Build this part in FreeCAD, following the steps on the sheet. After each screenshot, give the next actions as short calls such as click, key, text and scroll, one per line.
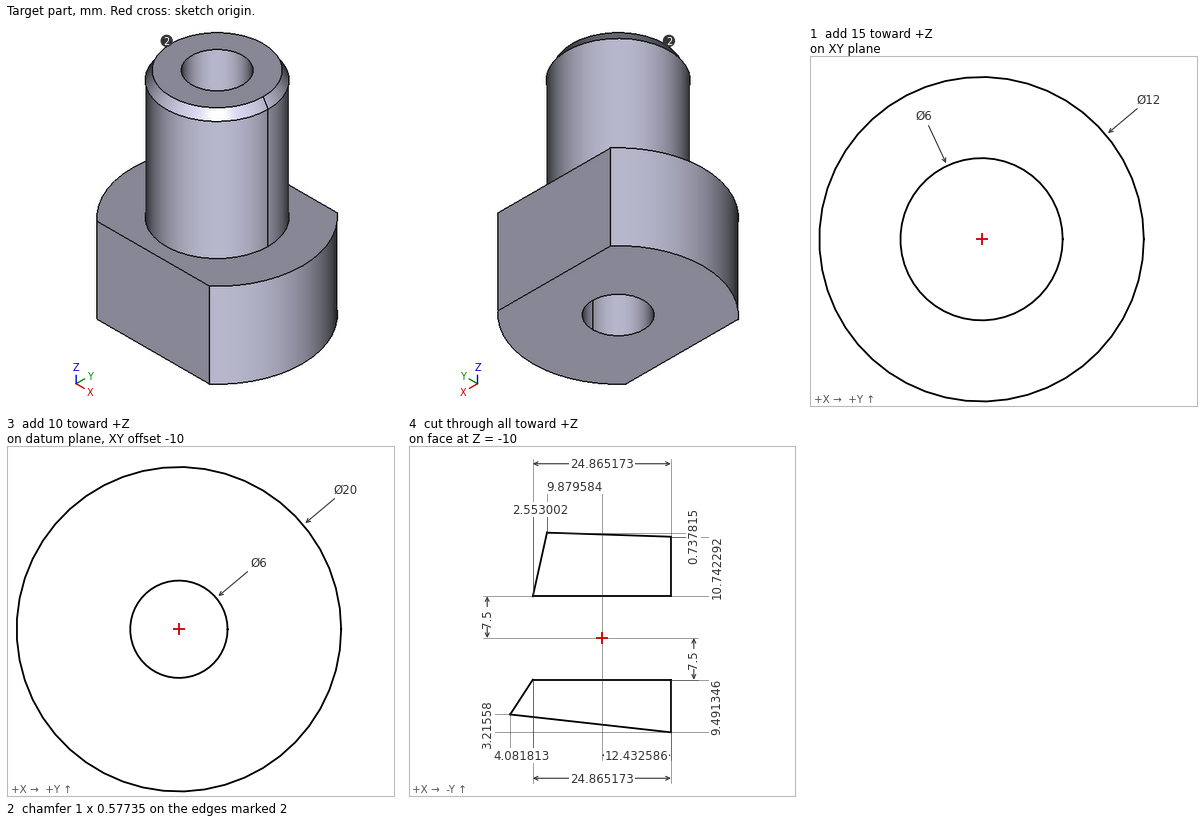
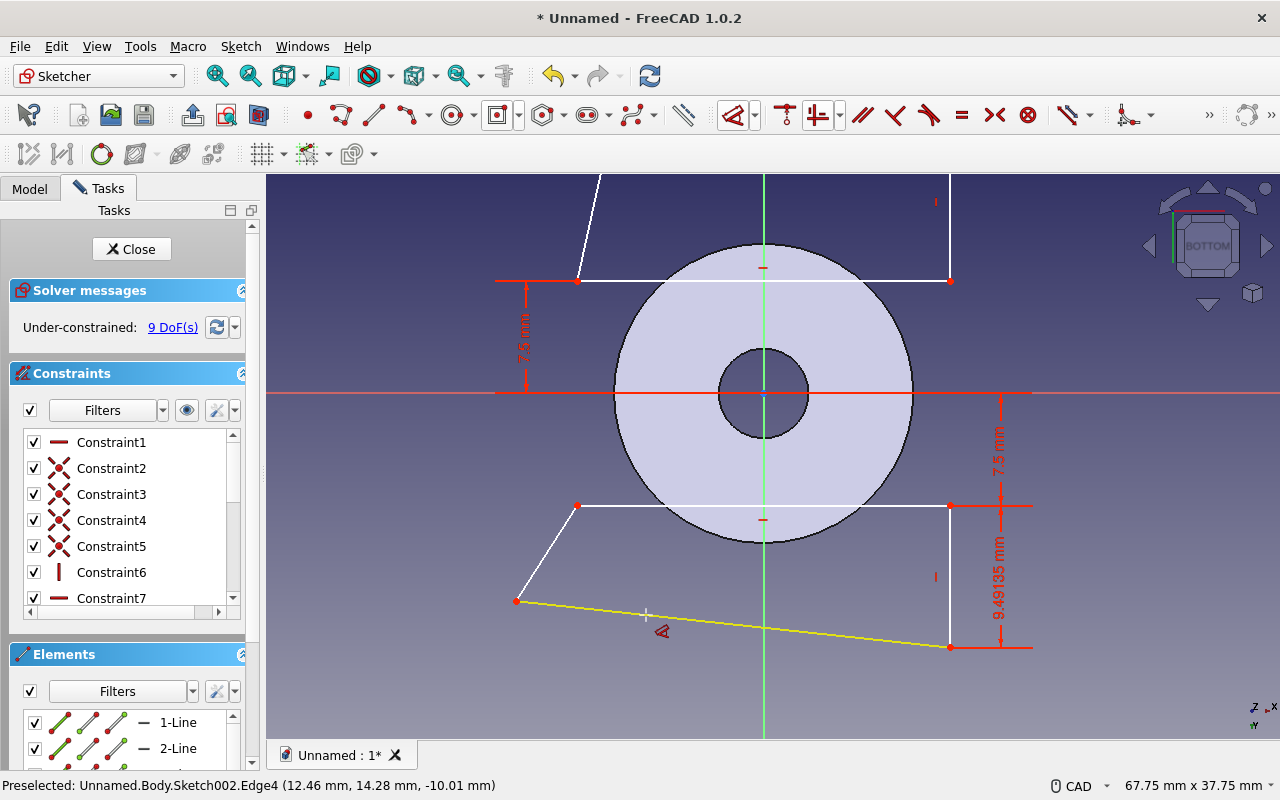
click(646, 615)
click(482, 624)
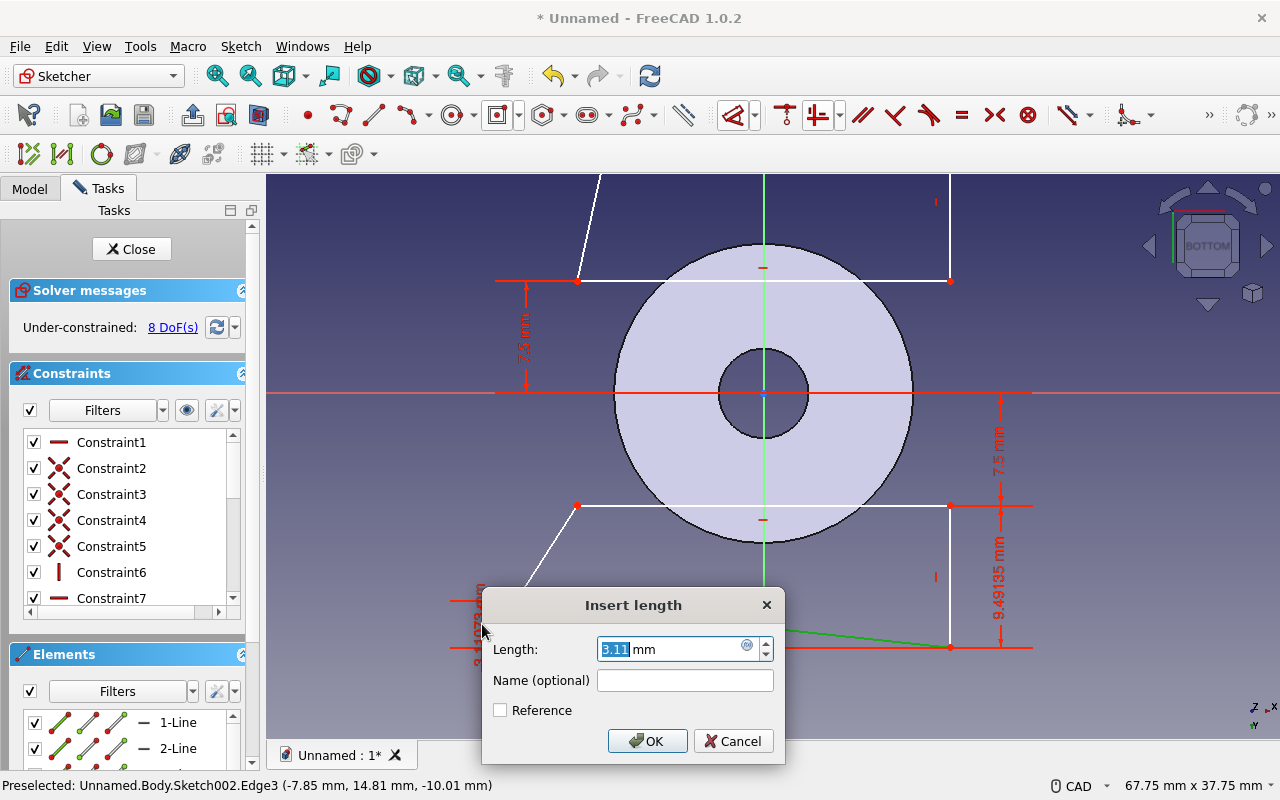
text(3.21558)
key(Return)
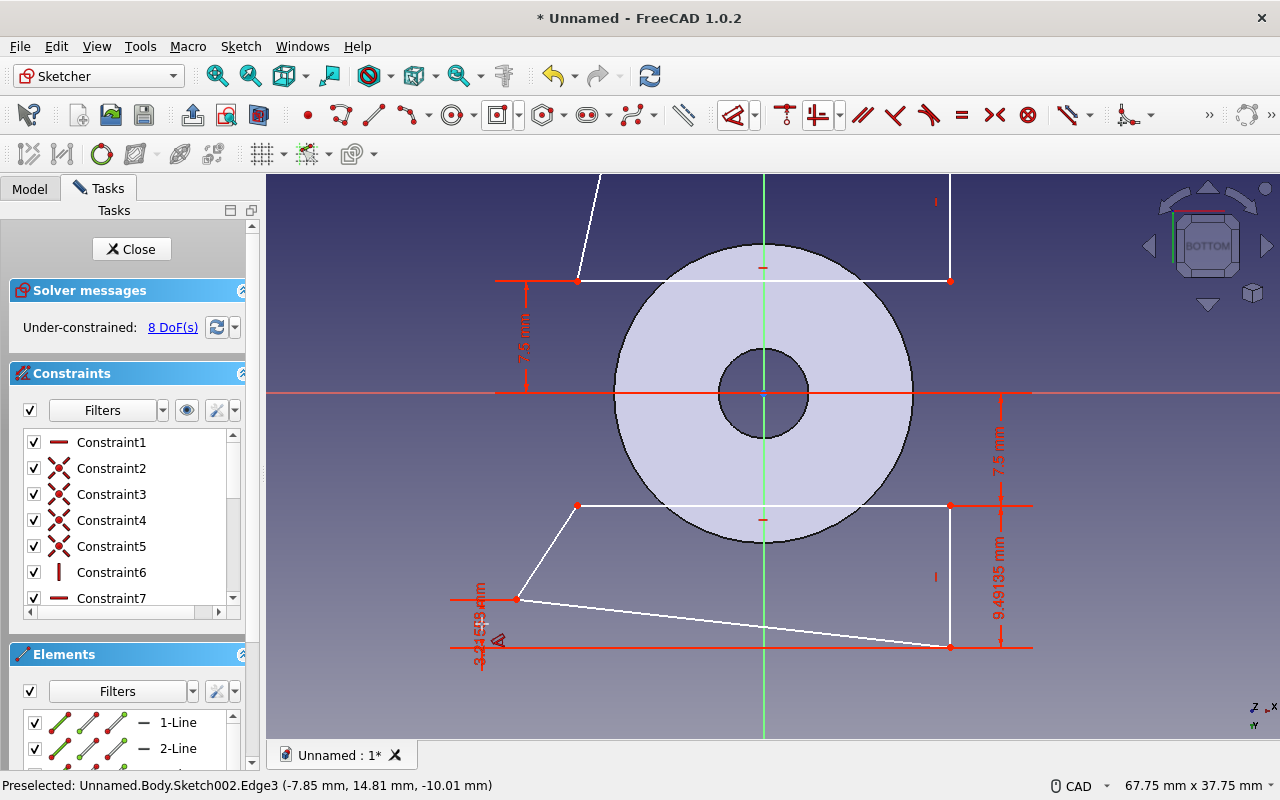
click(838, 506)
click(678, 540)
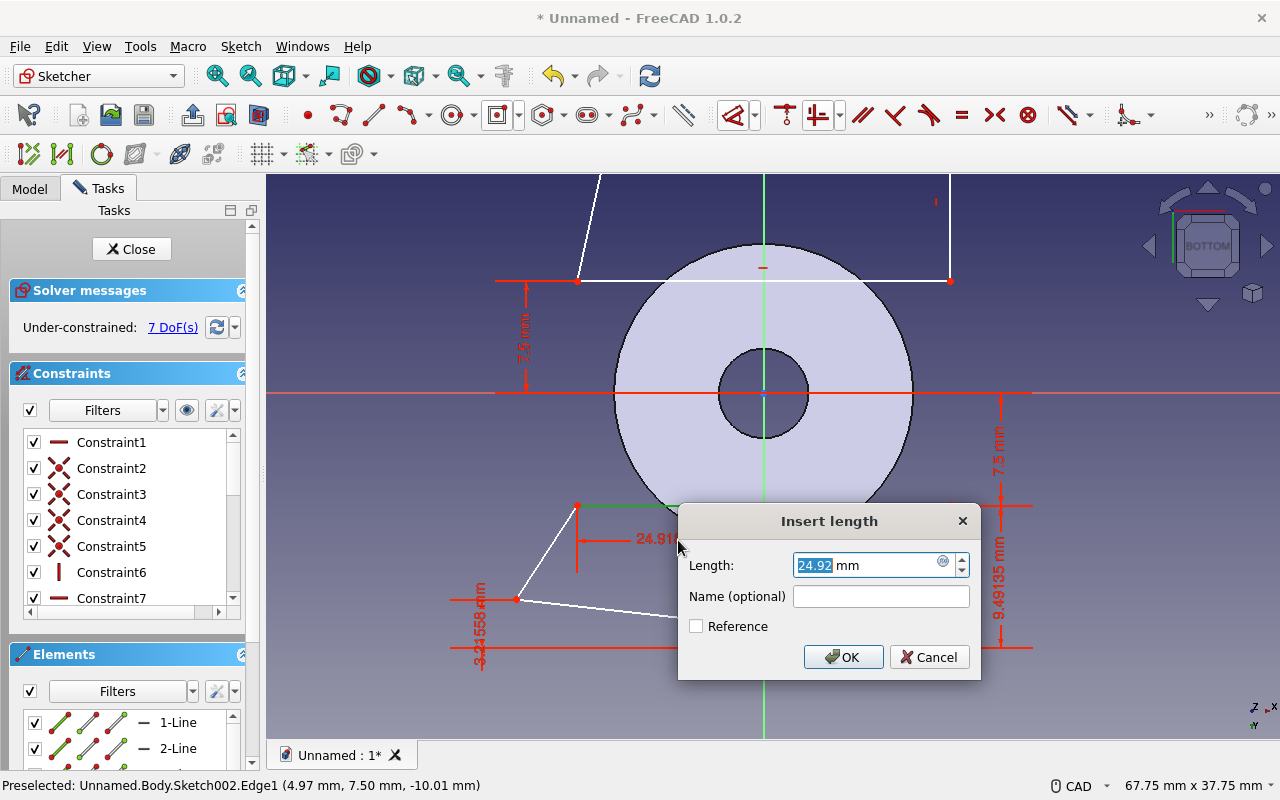
text(24.865173)
key(Return)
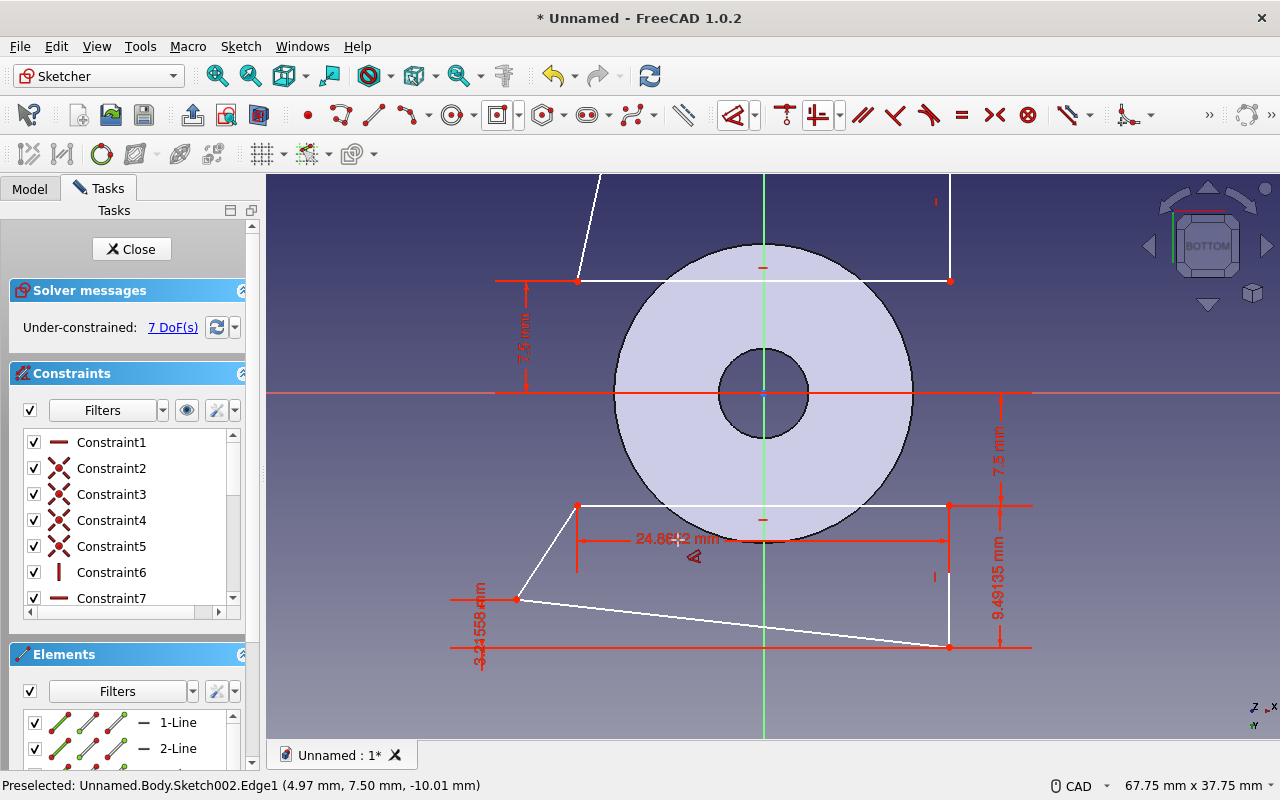
click(689, 281)
click(678, 247)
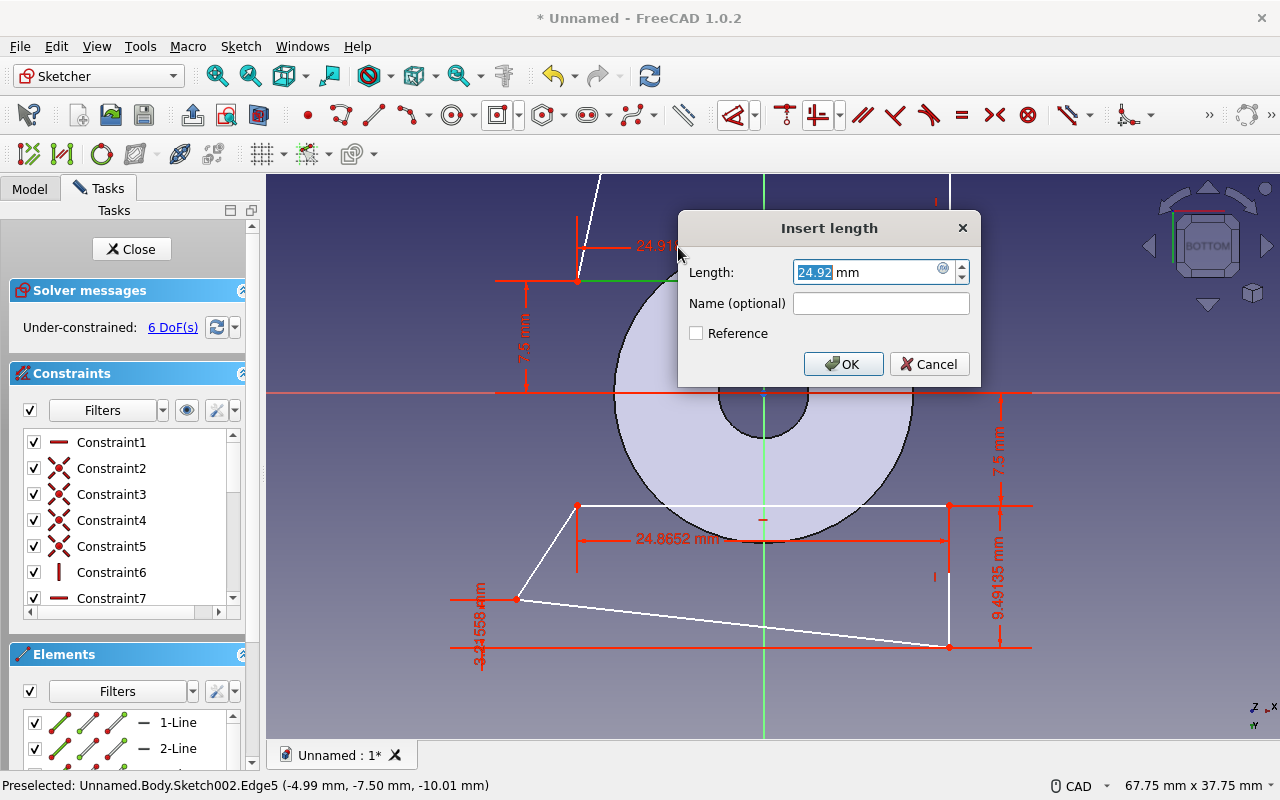
text(24.865173)
key(Return)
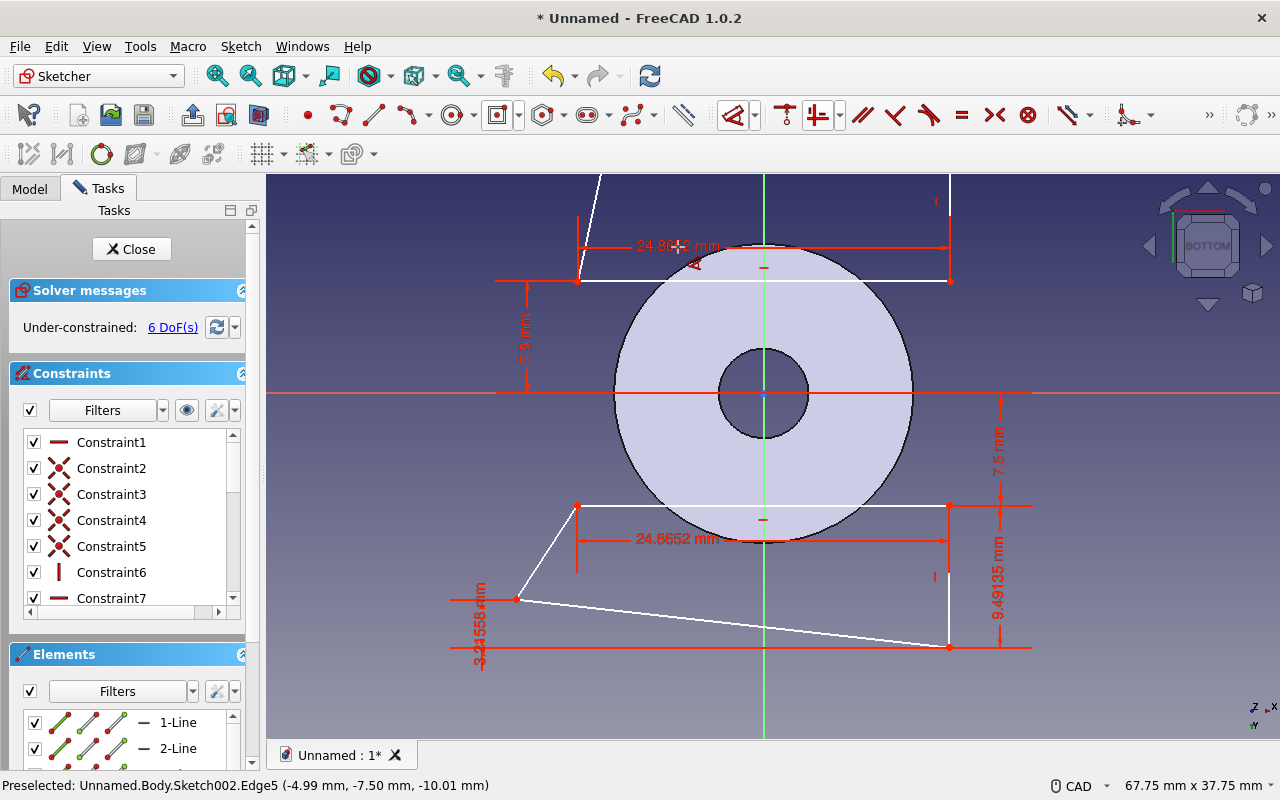
click(950, 234)
click(984, 242)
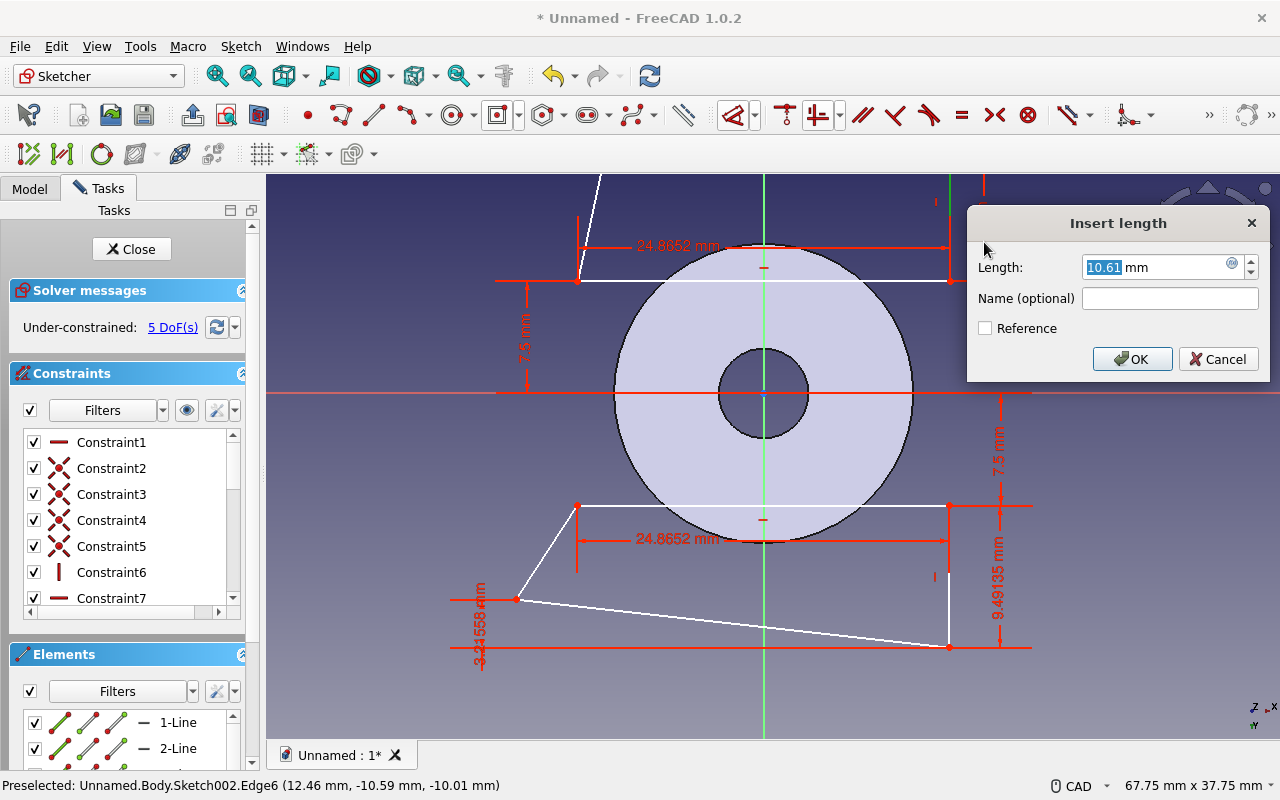
text(10.742292)
key(Return)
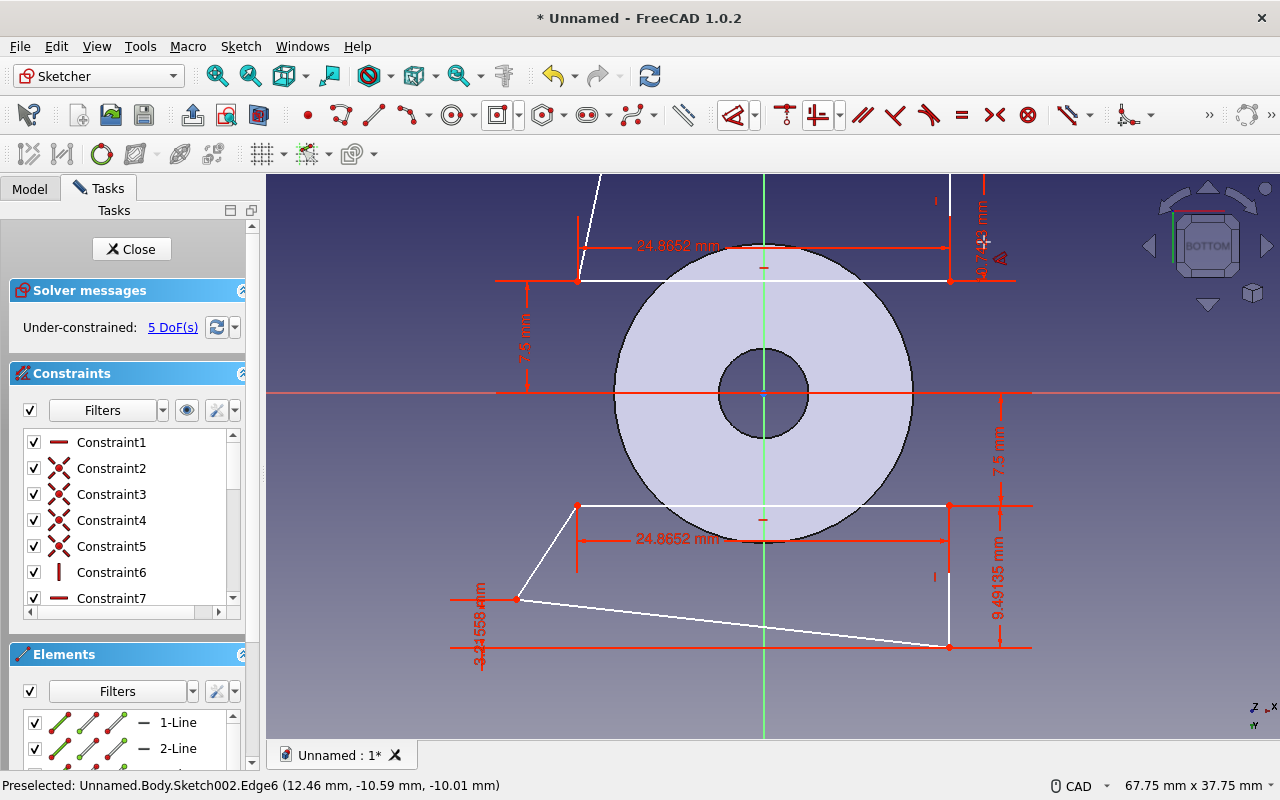
scroll(646, 615, down, 2)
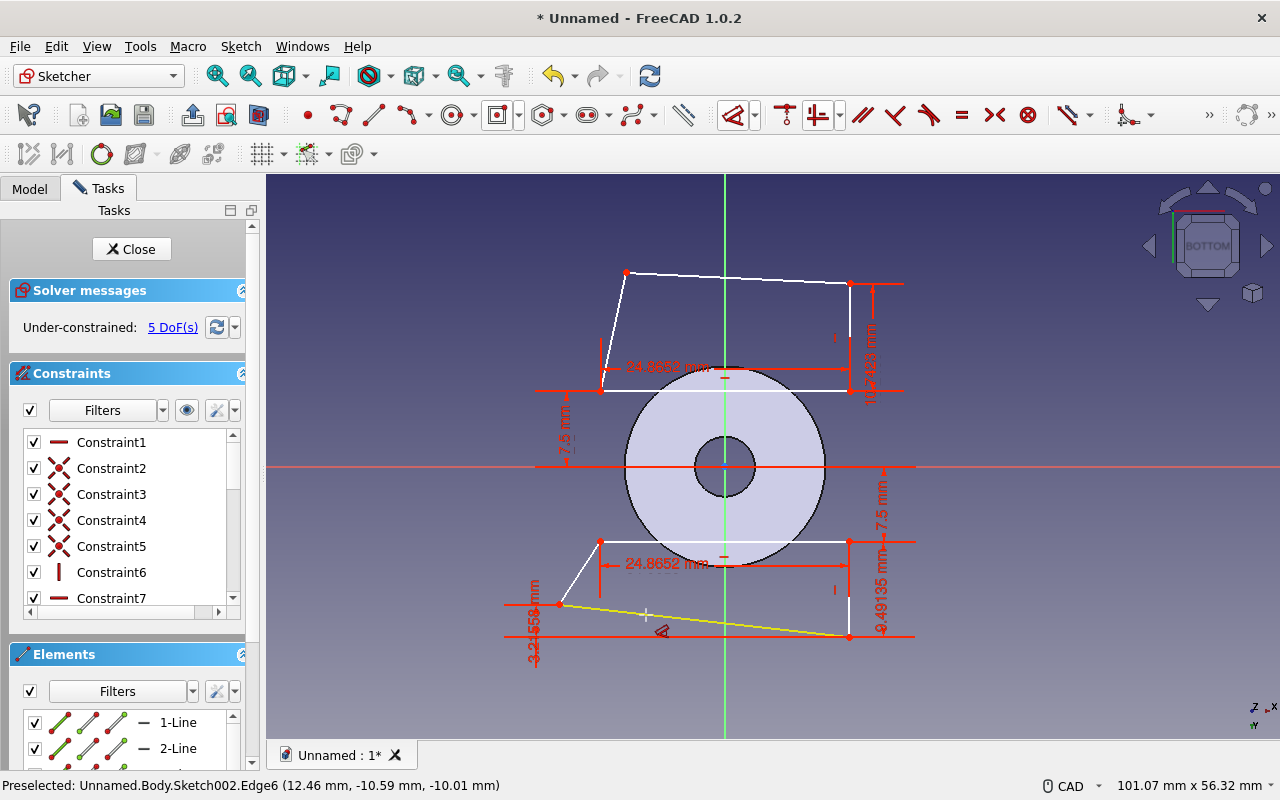
click(626, 273)
click(675, 239)